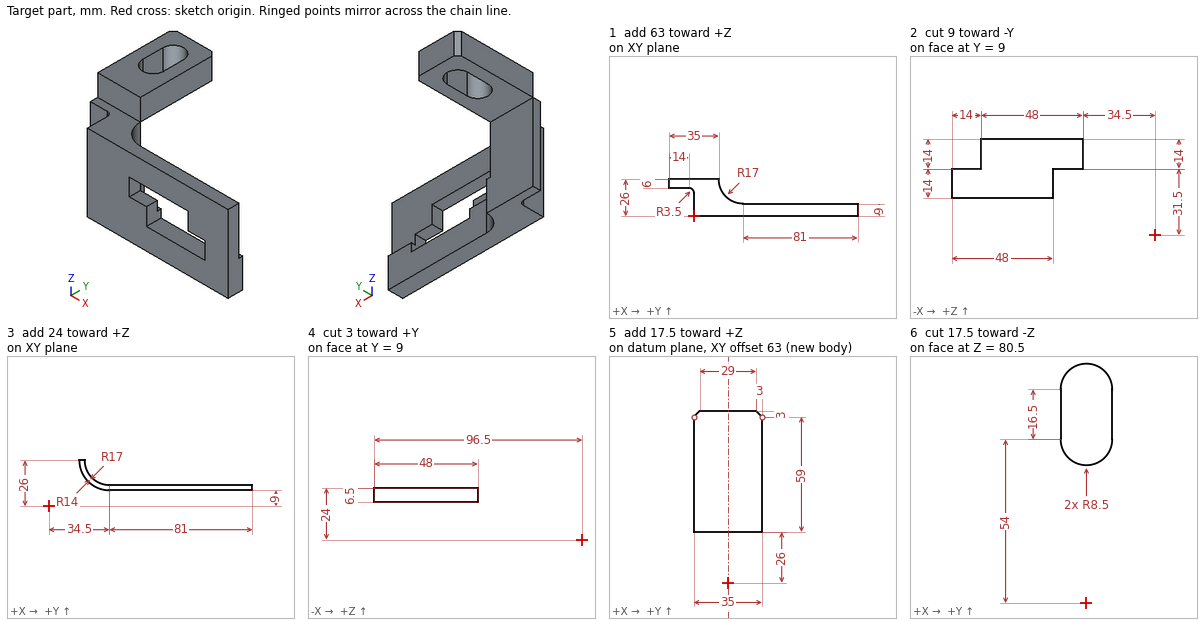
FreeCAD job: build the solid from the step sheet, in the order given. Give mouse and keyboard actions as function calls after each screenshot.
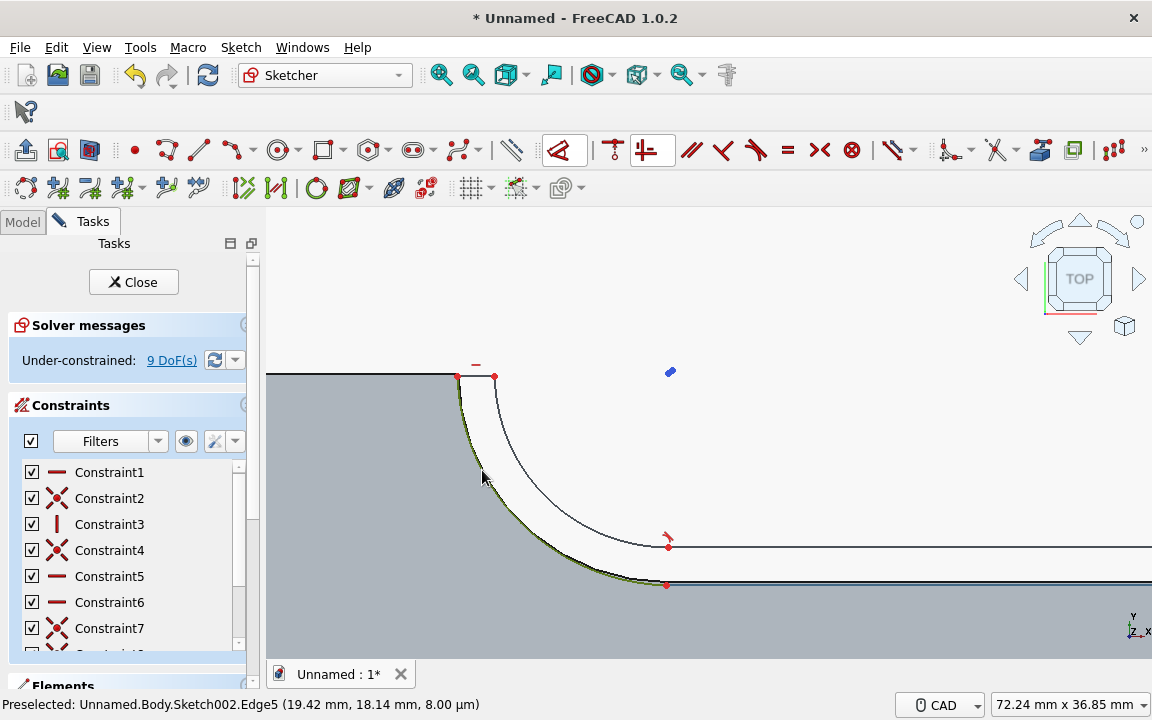
key(t)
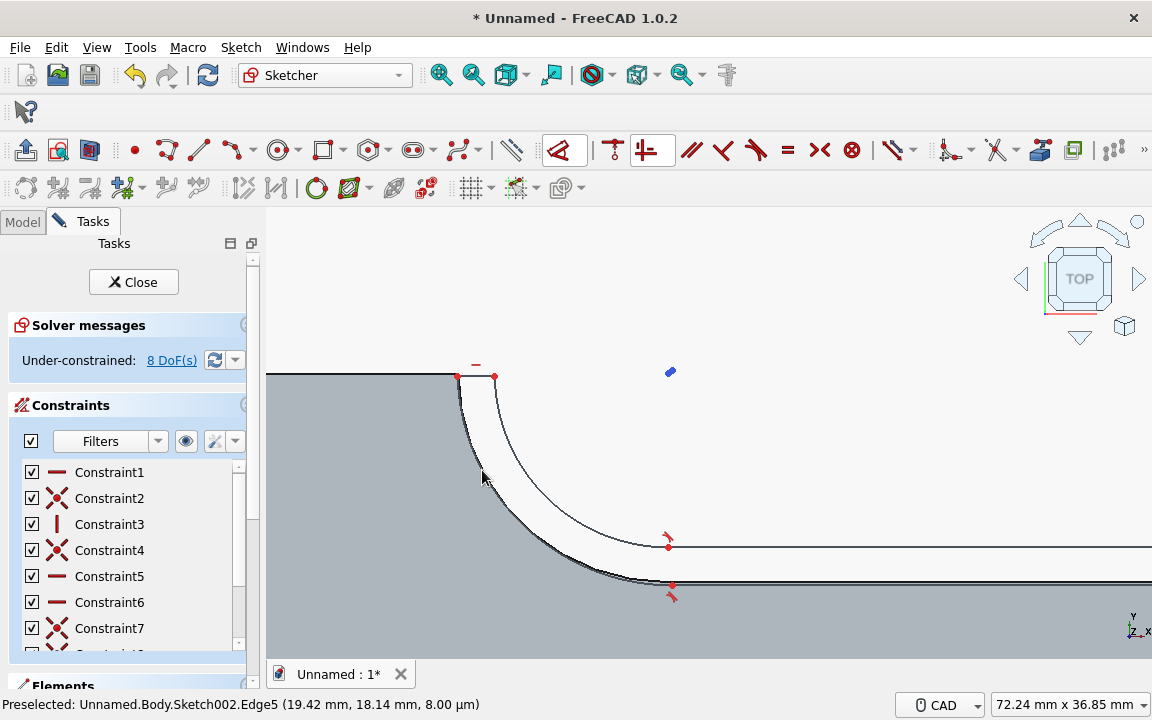
click(483, 472)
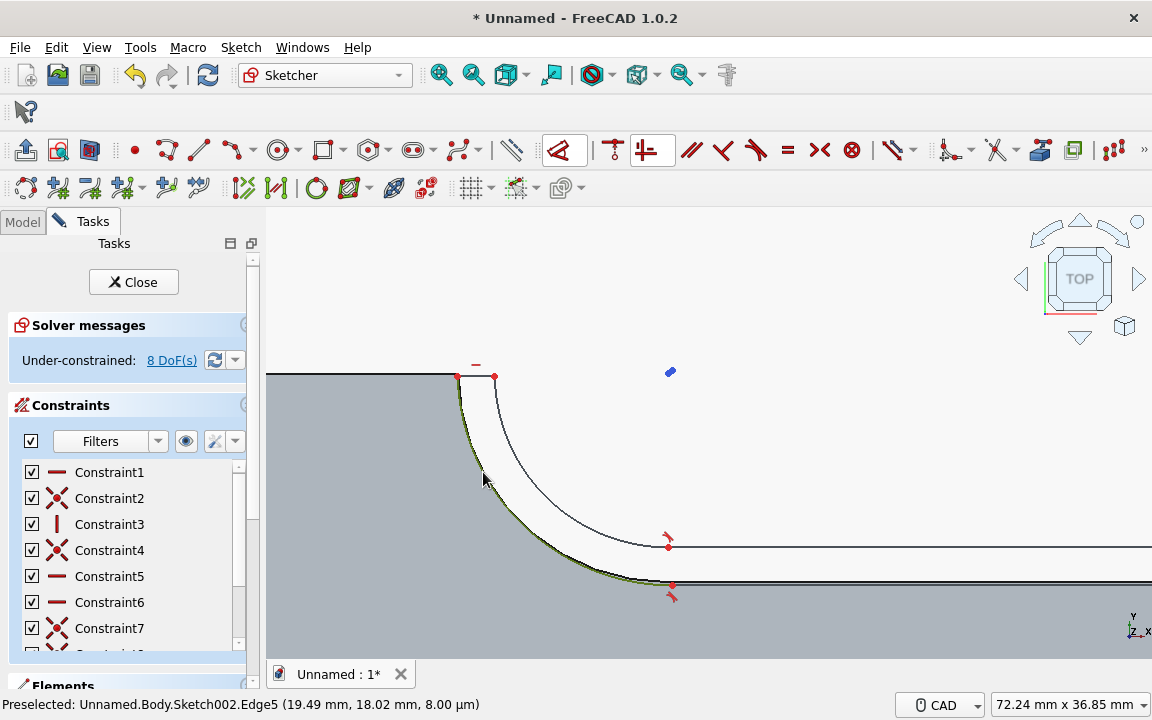
click(514, 454)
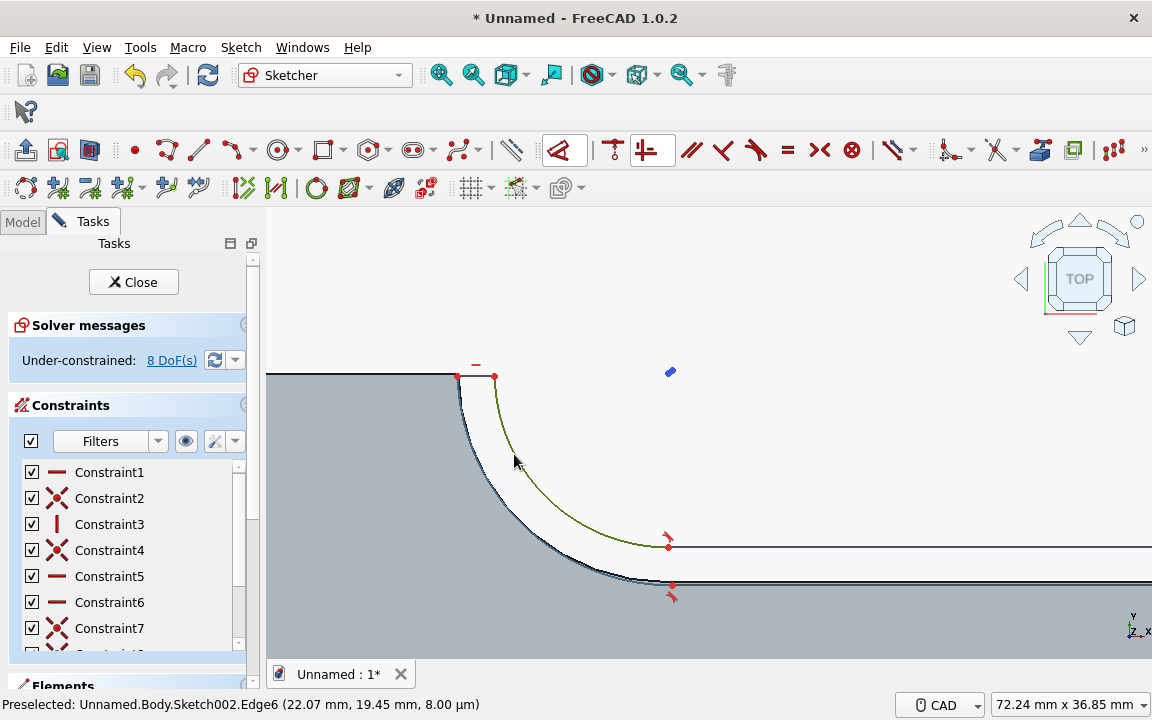
key(c)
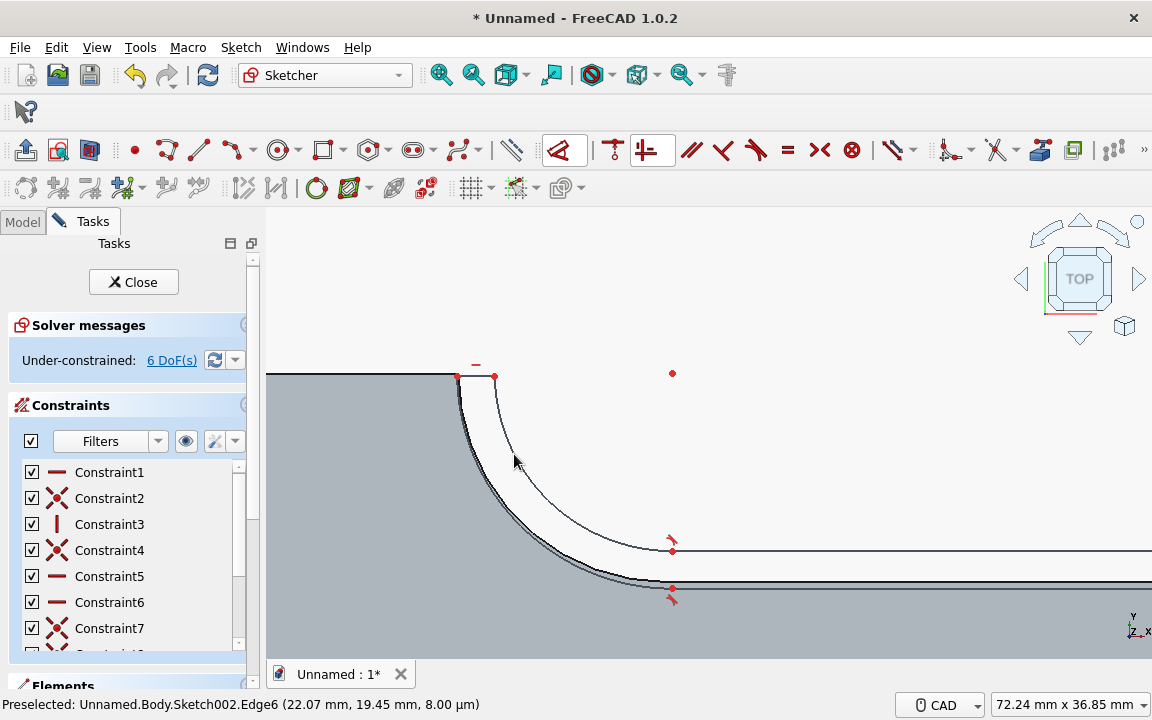
click(482, 473)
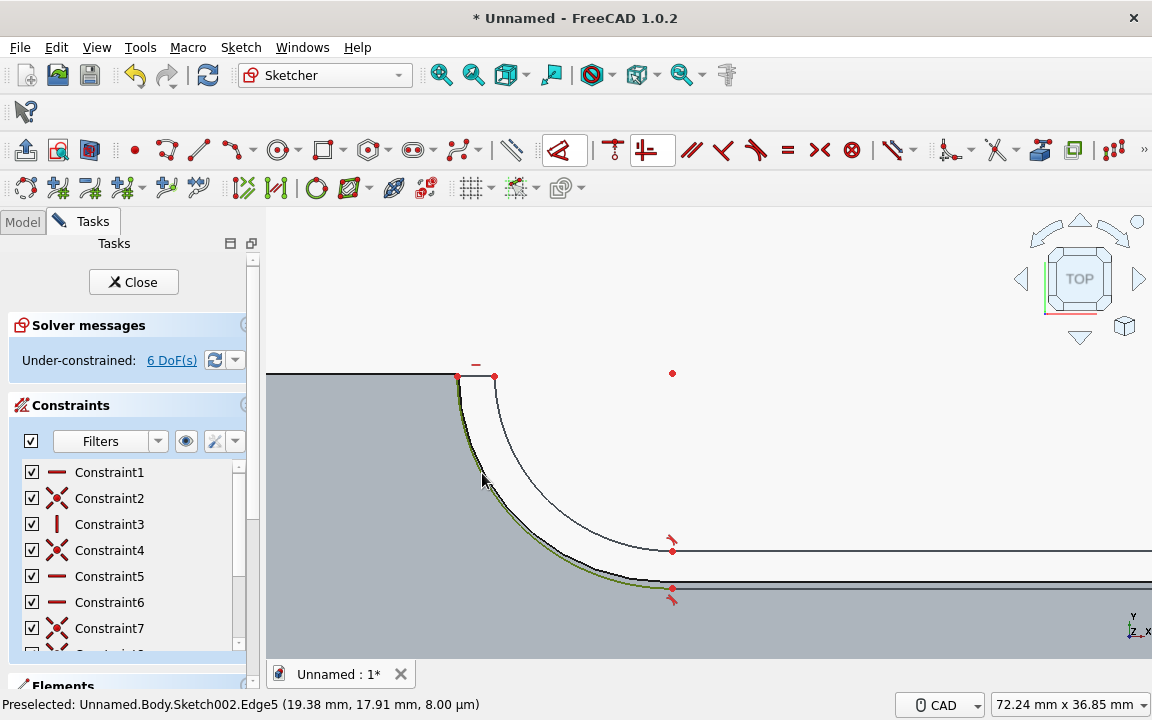
key(k)
key(r)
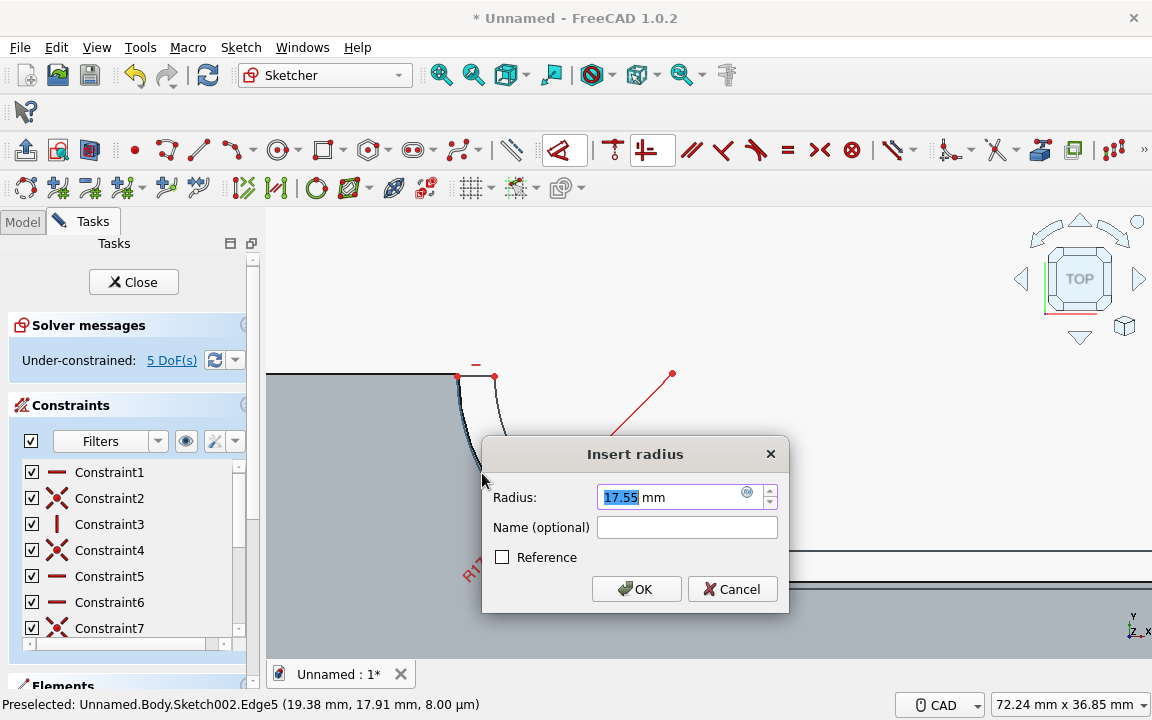
text(17)
key(Return)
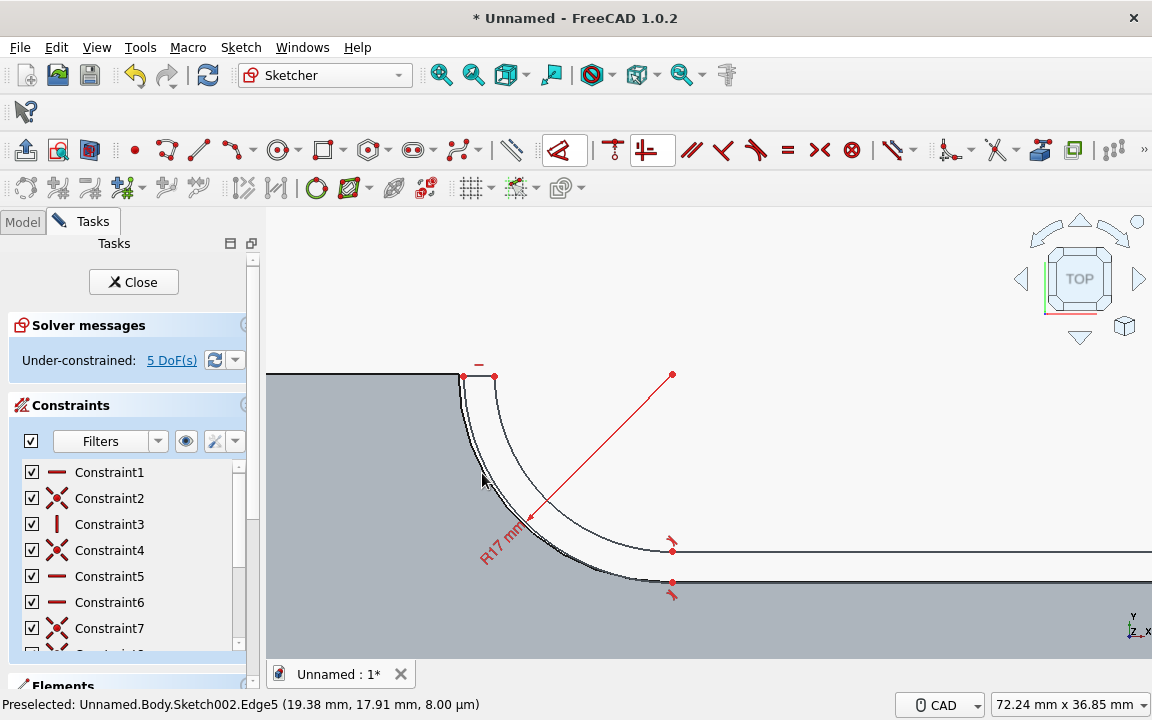
click(515, 456)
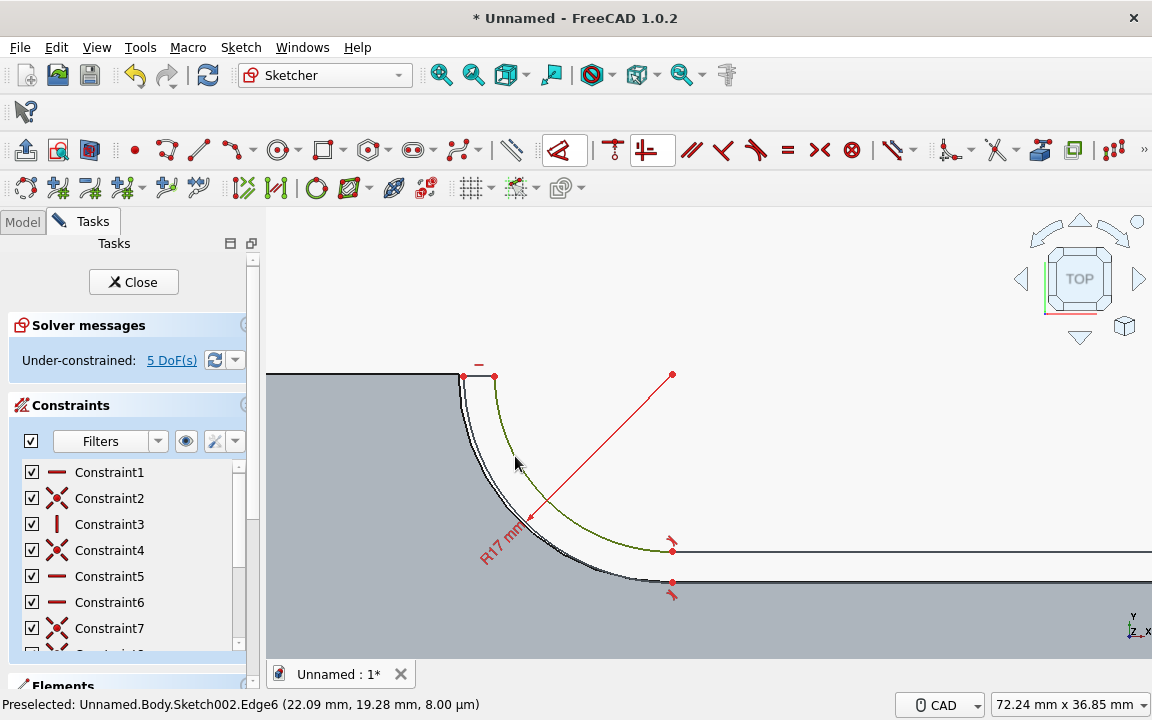
click(582, 150)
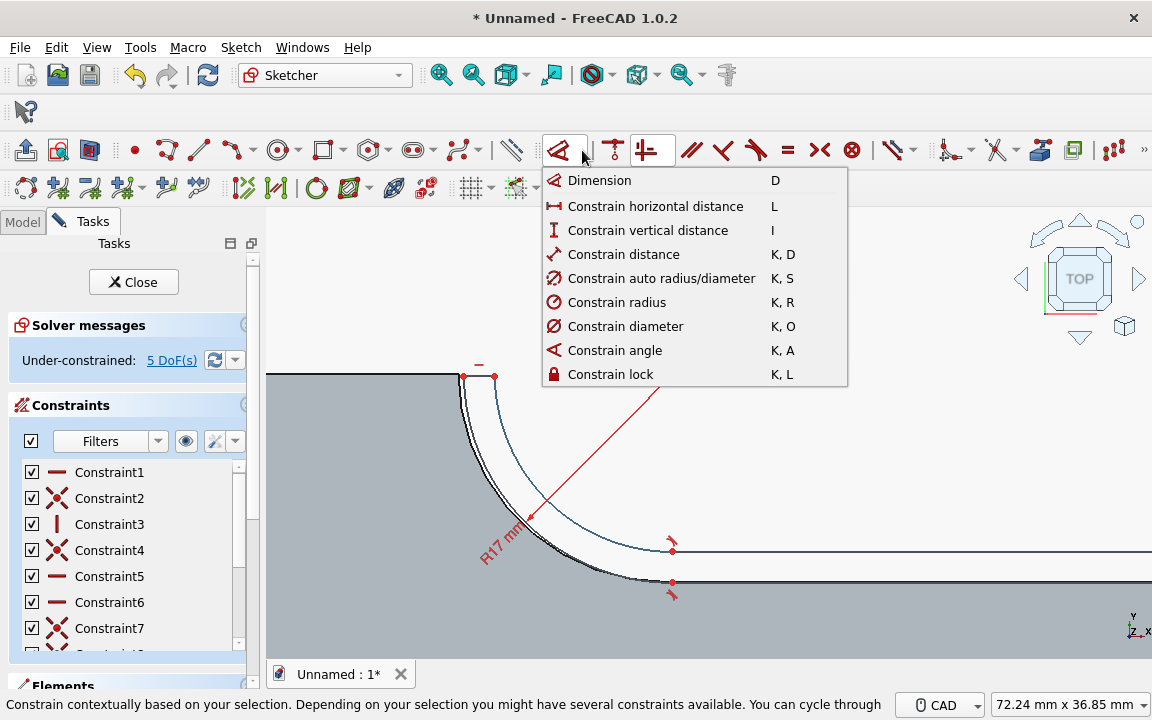
click(695, 302)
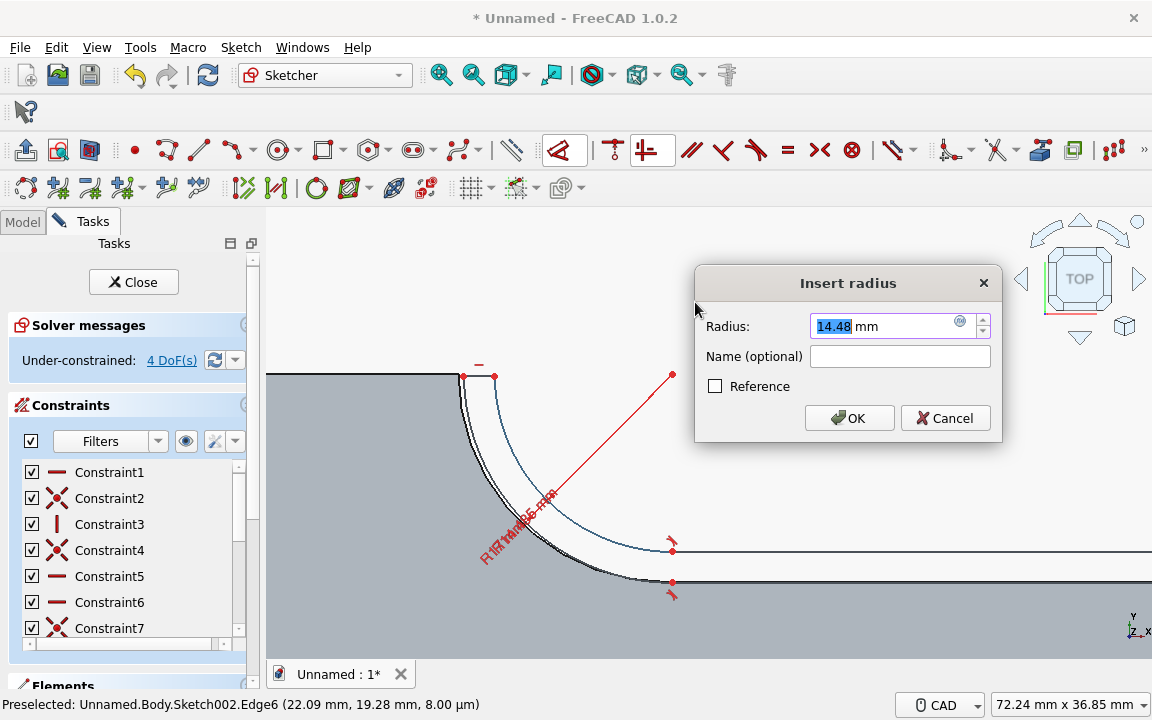
text(14)
key(Return)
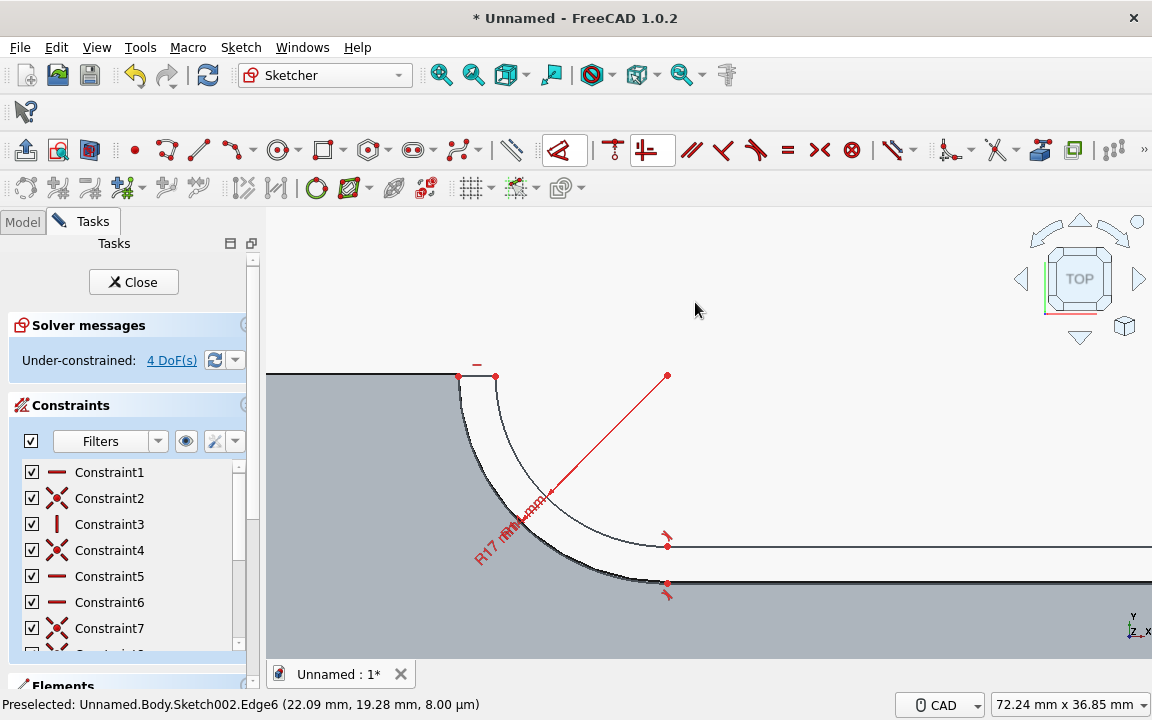
click(965, 547)